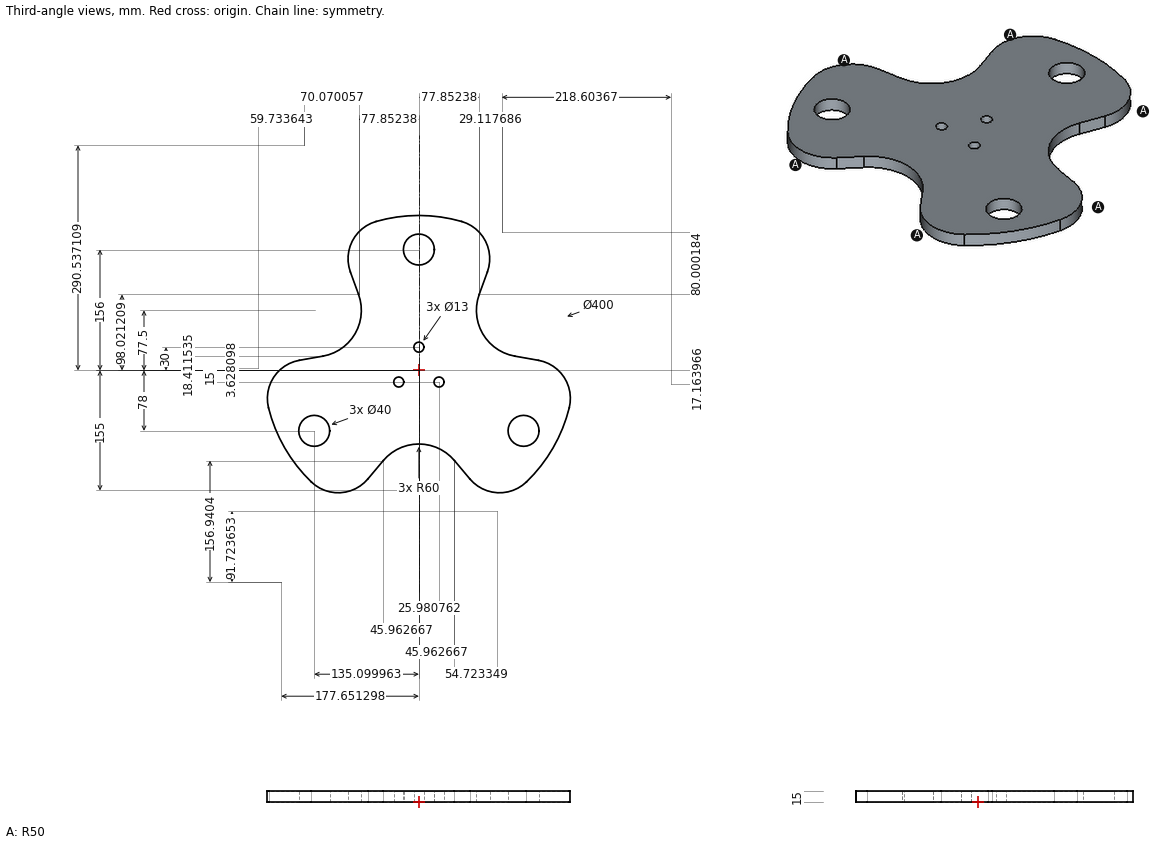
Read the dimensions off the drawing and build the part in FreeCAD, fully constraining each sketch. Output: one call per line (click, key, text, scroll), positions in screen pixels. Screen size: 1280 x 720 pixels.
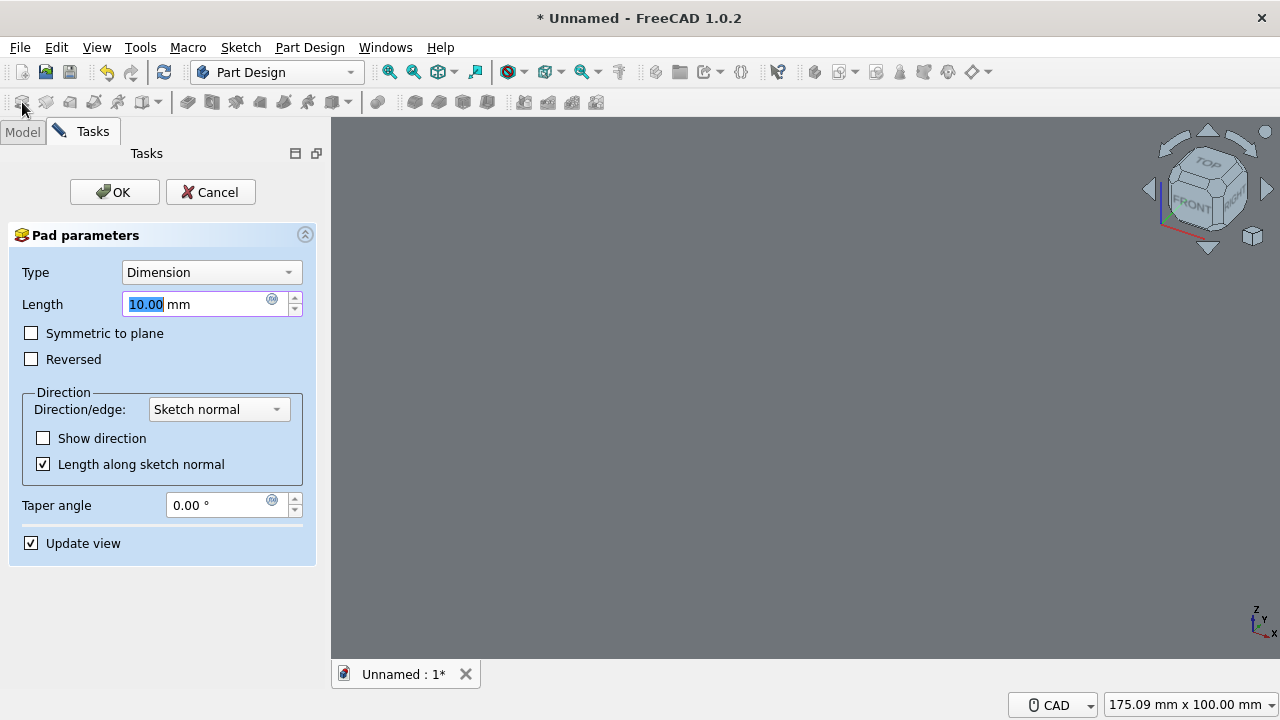
text(15)
key(Tab)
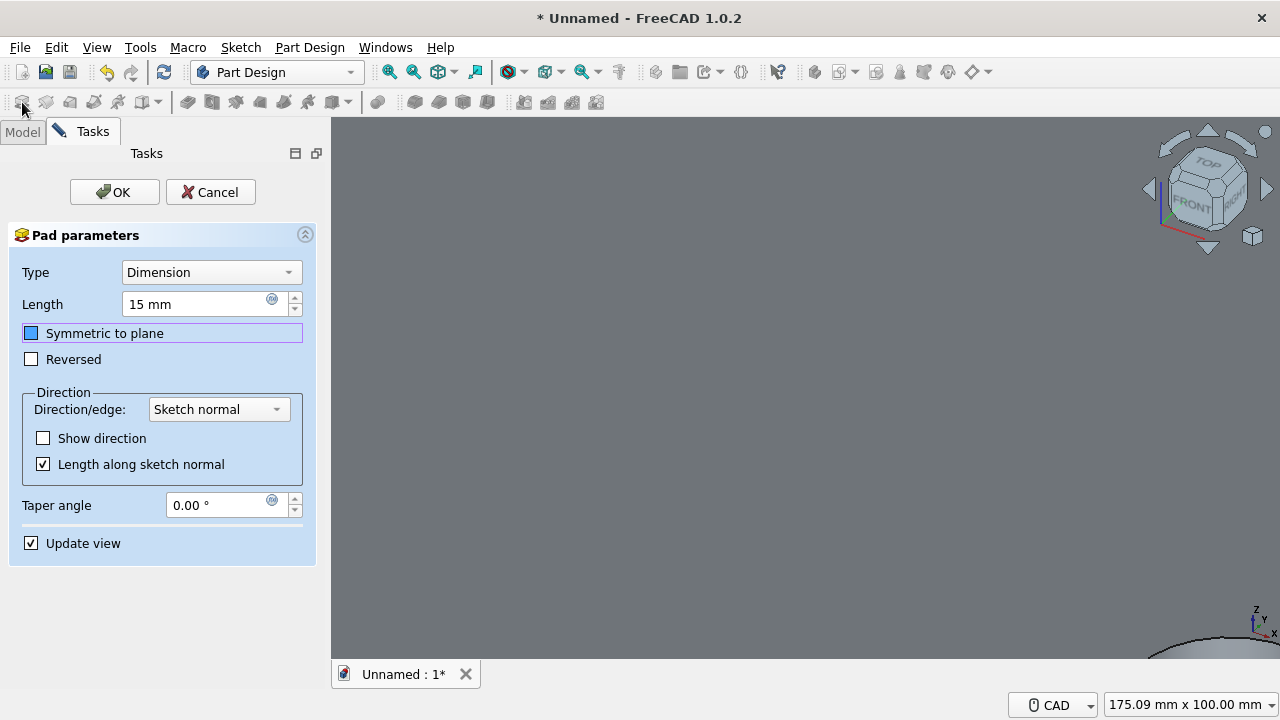
click(115, 192)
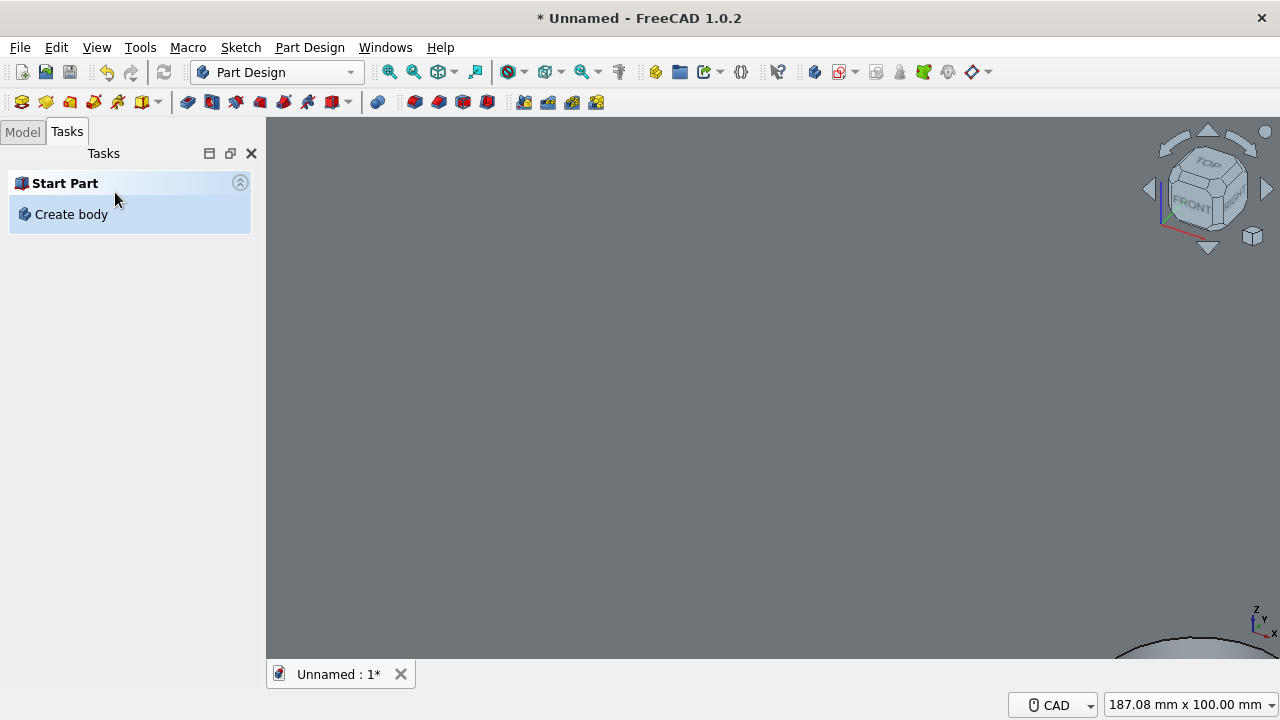
click(390, 72)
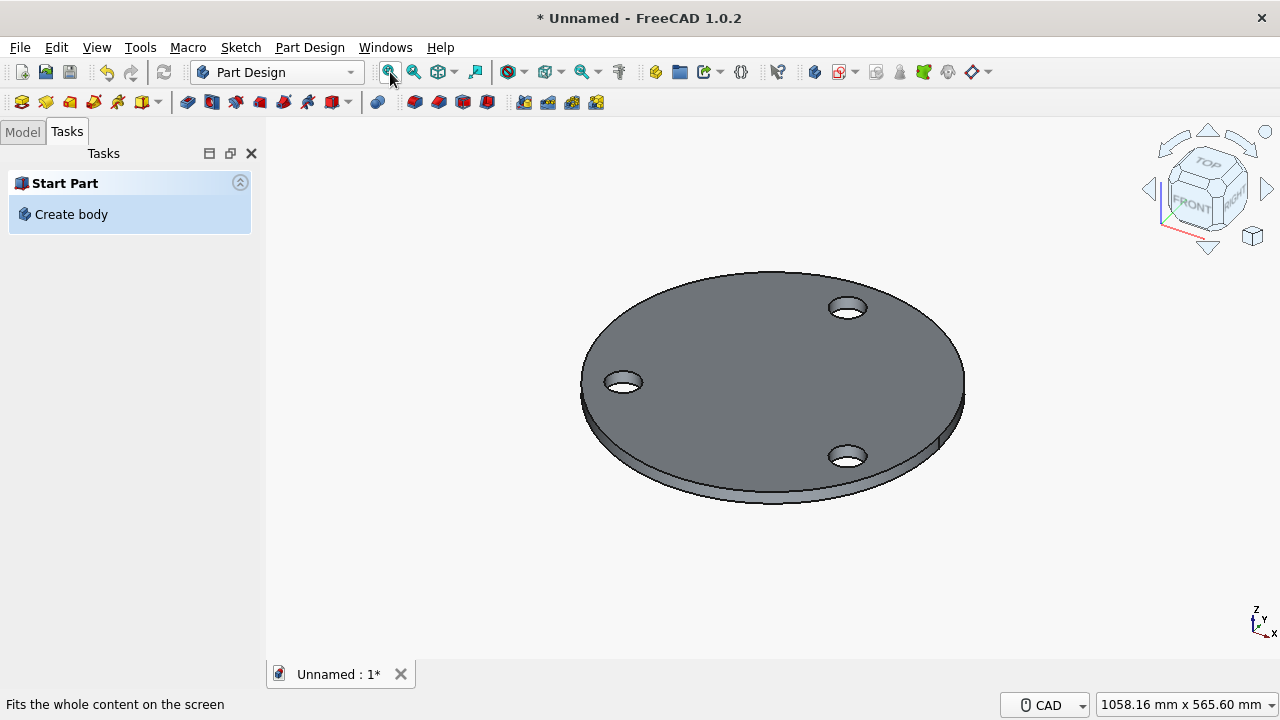
click(773, 381)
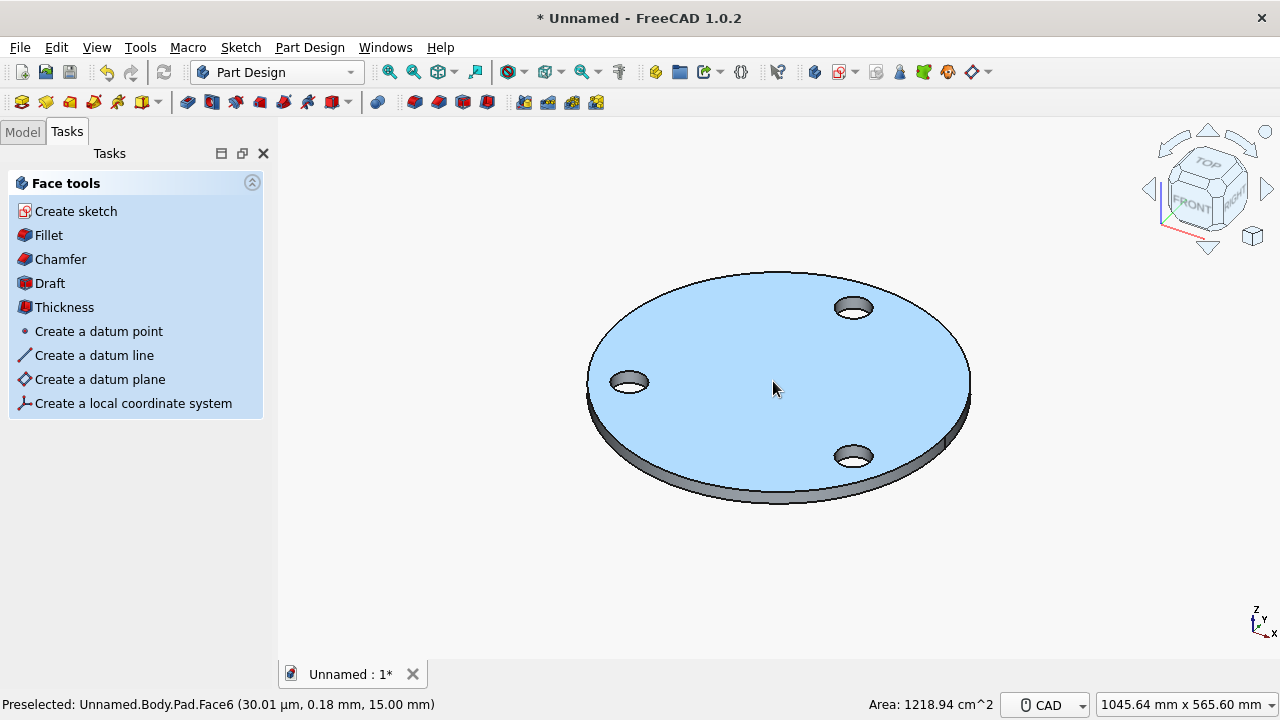
click(840, 72)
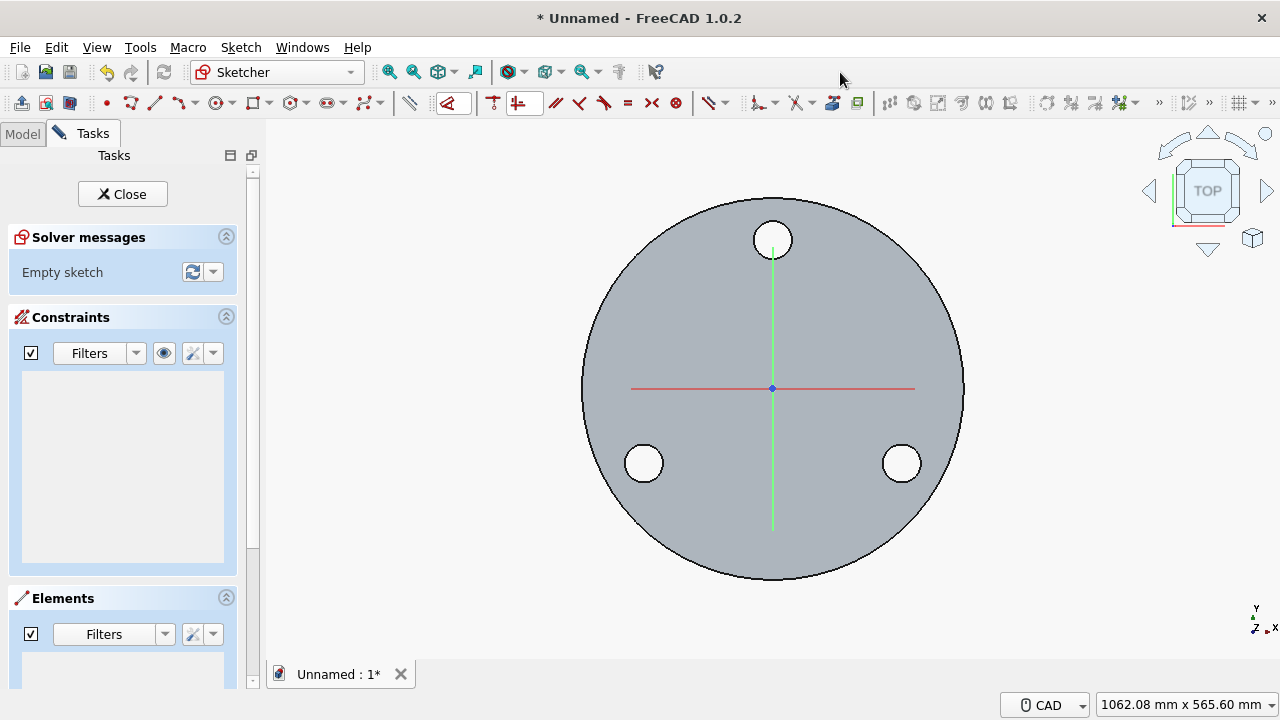
scroll(451, 406, down, 2)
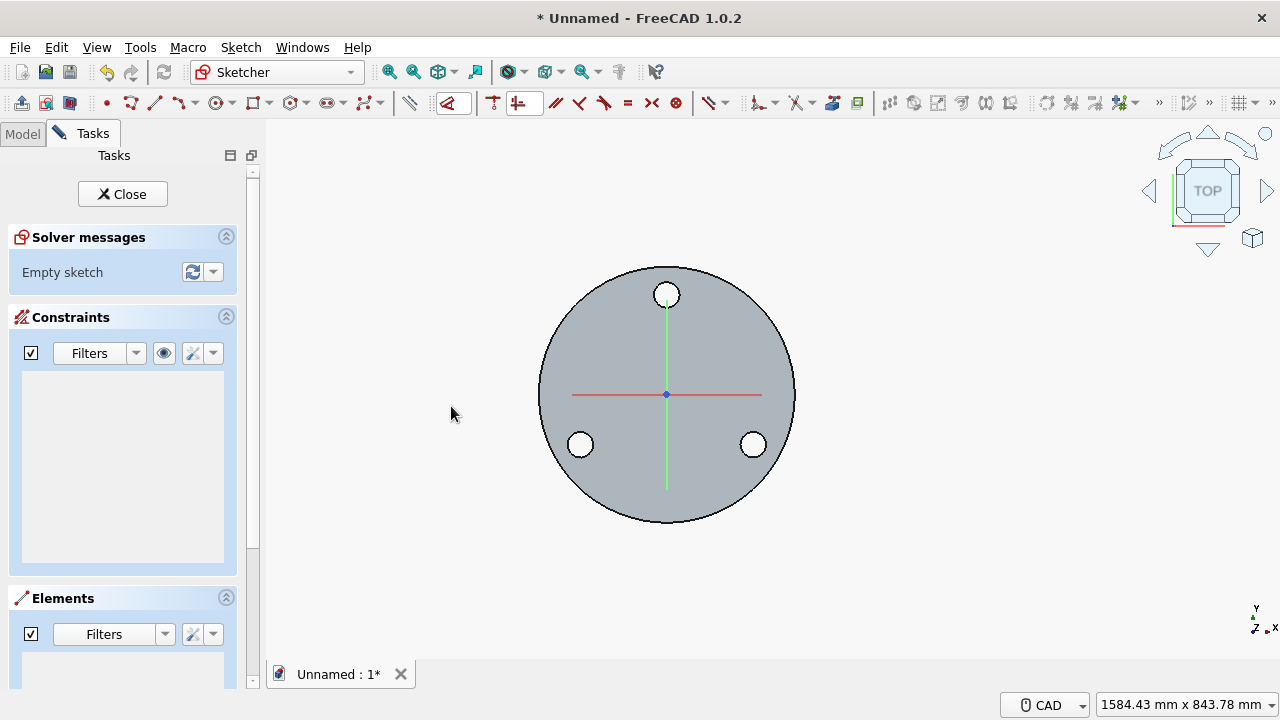
click(132, 104)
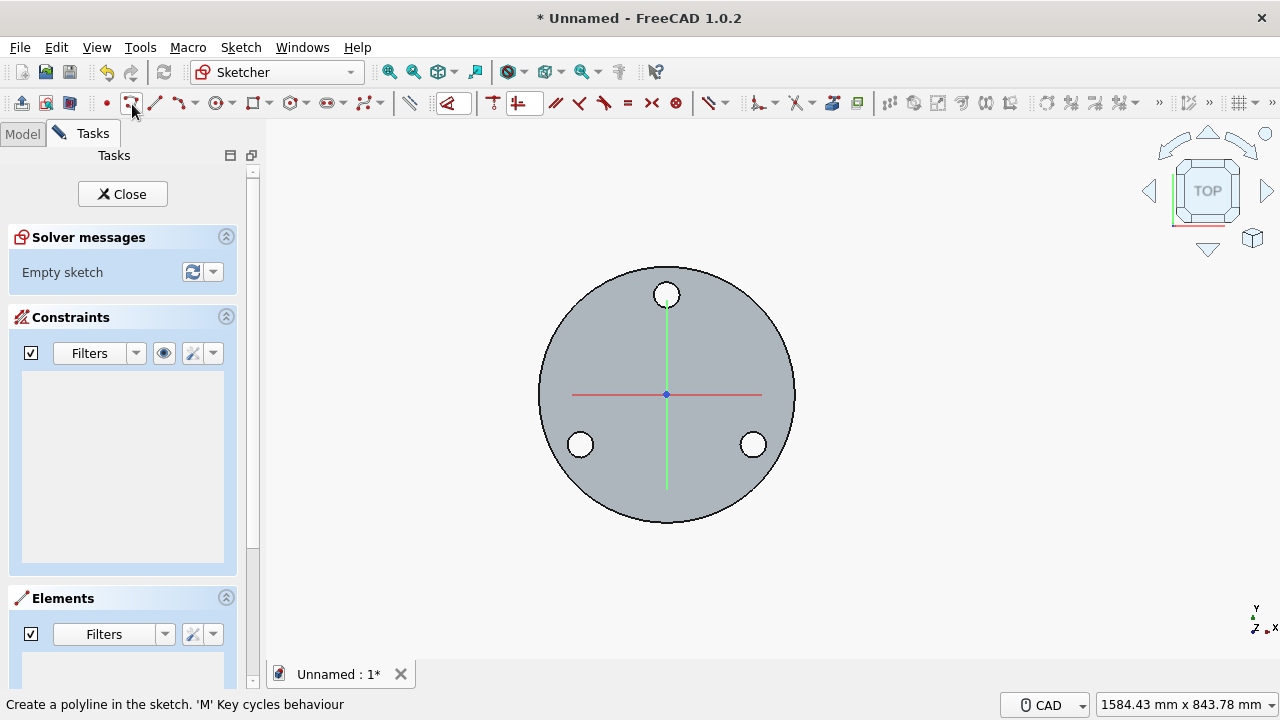
click(637, 469)
click(553, 570)
click(731, 511)
click(696, 469)
right_click(696, 469)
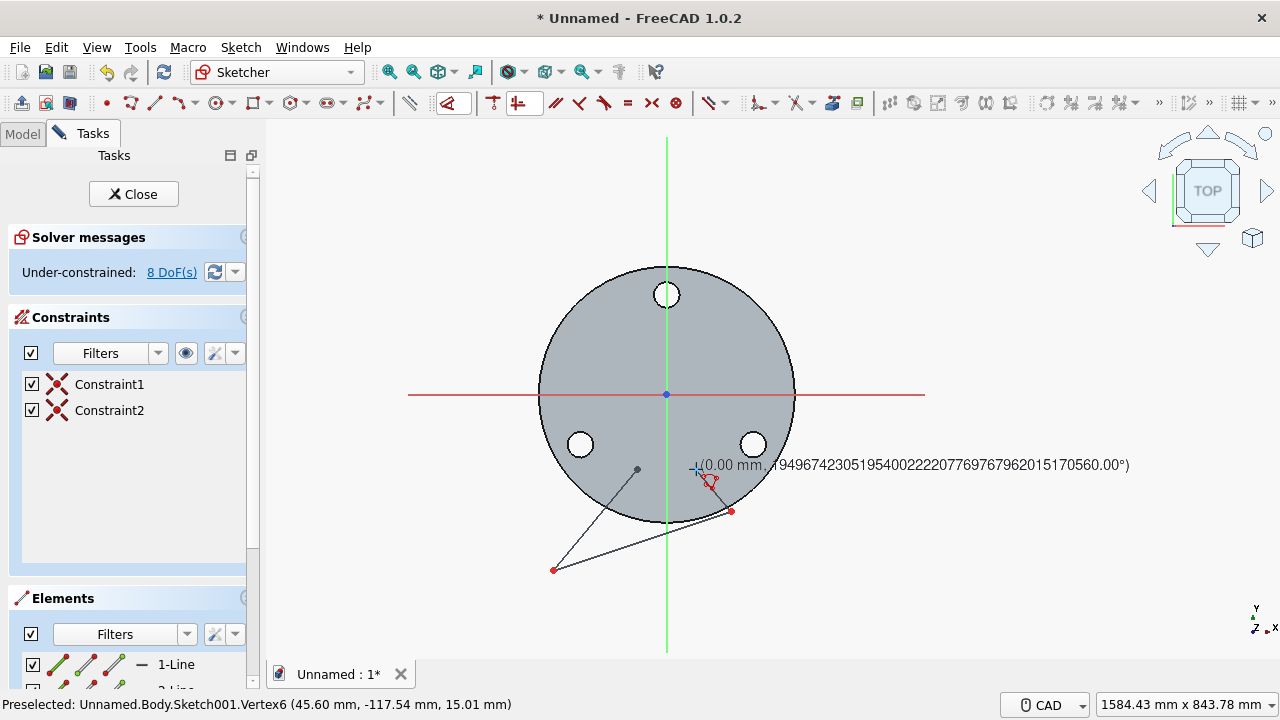
click(180, 104)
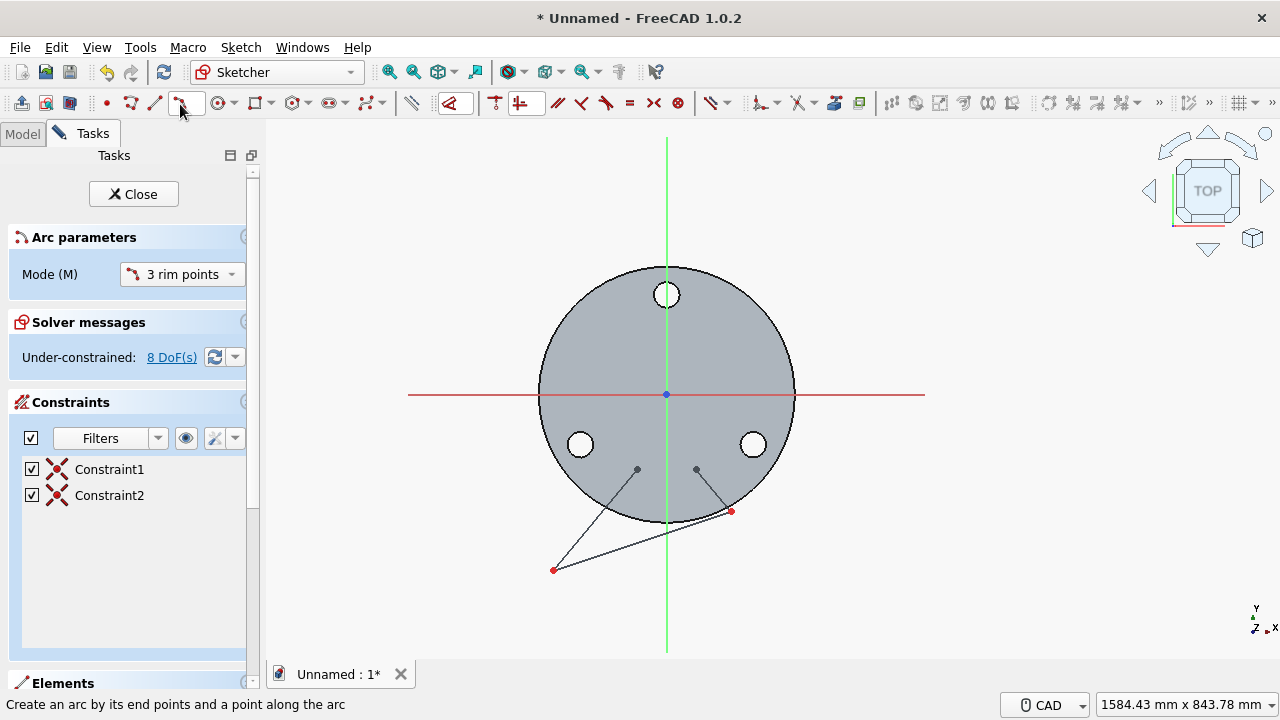
click(696, 470)
click(637, 470)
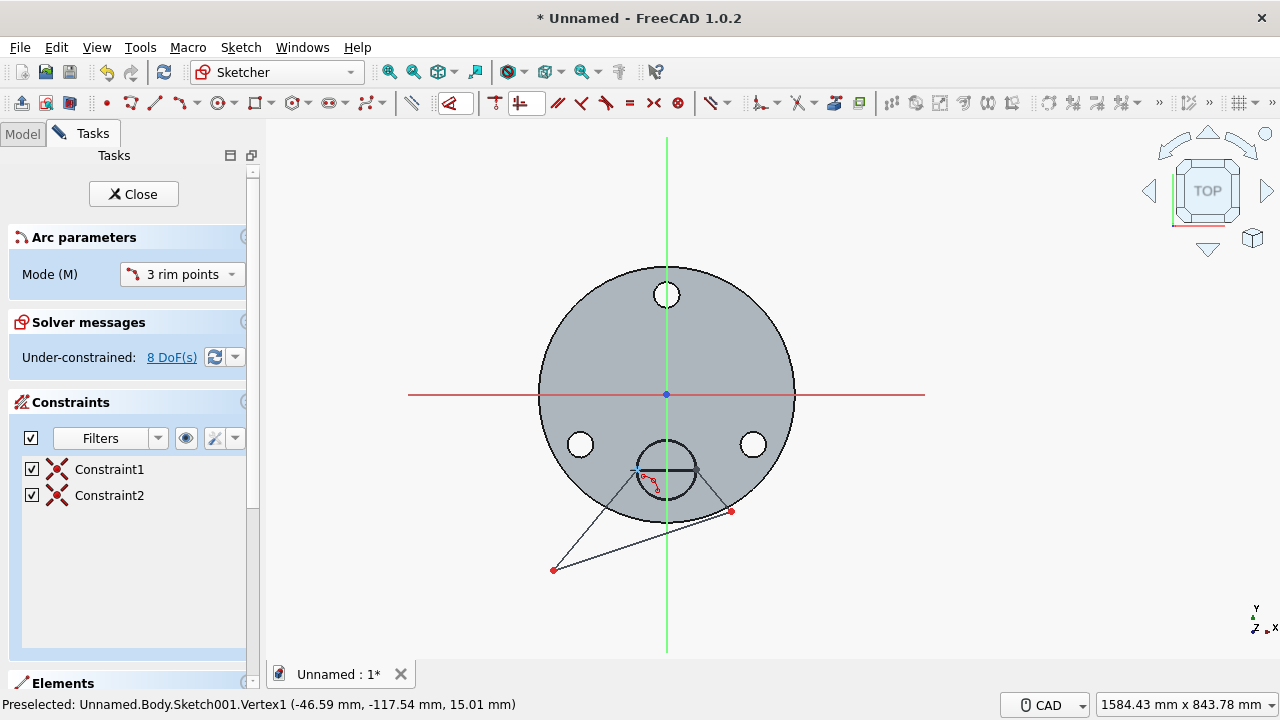
scroll(680, 458, up, 2)